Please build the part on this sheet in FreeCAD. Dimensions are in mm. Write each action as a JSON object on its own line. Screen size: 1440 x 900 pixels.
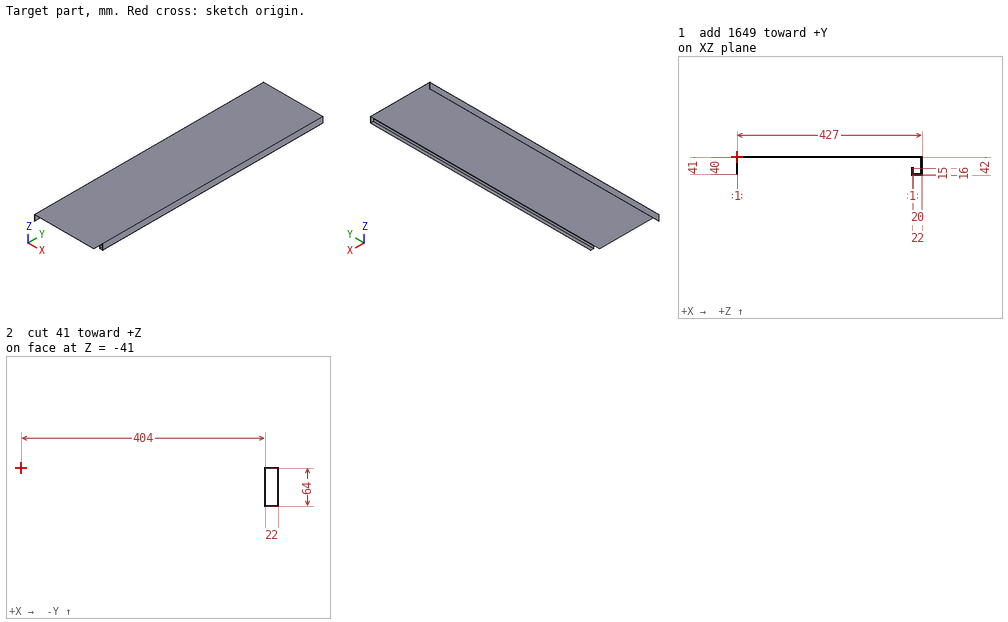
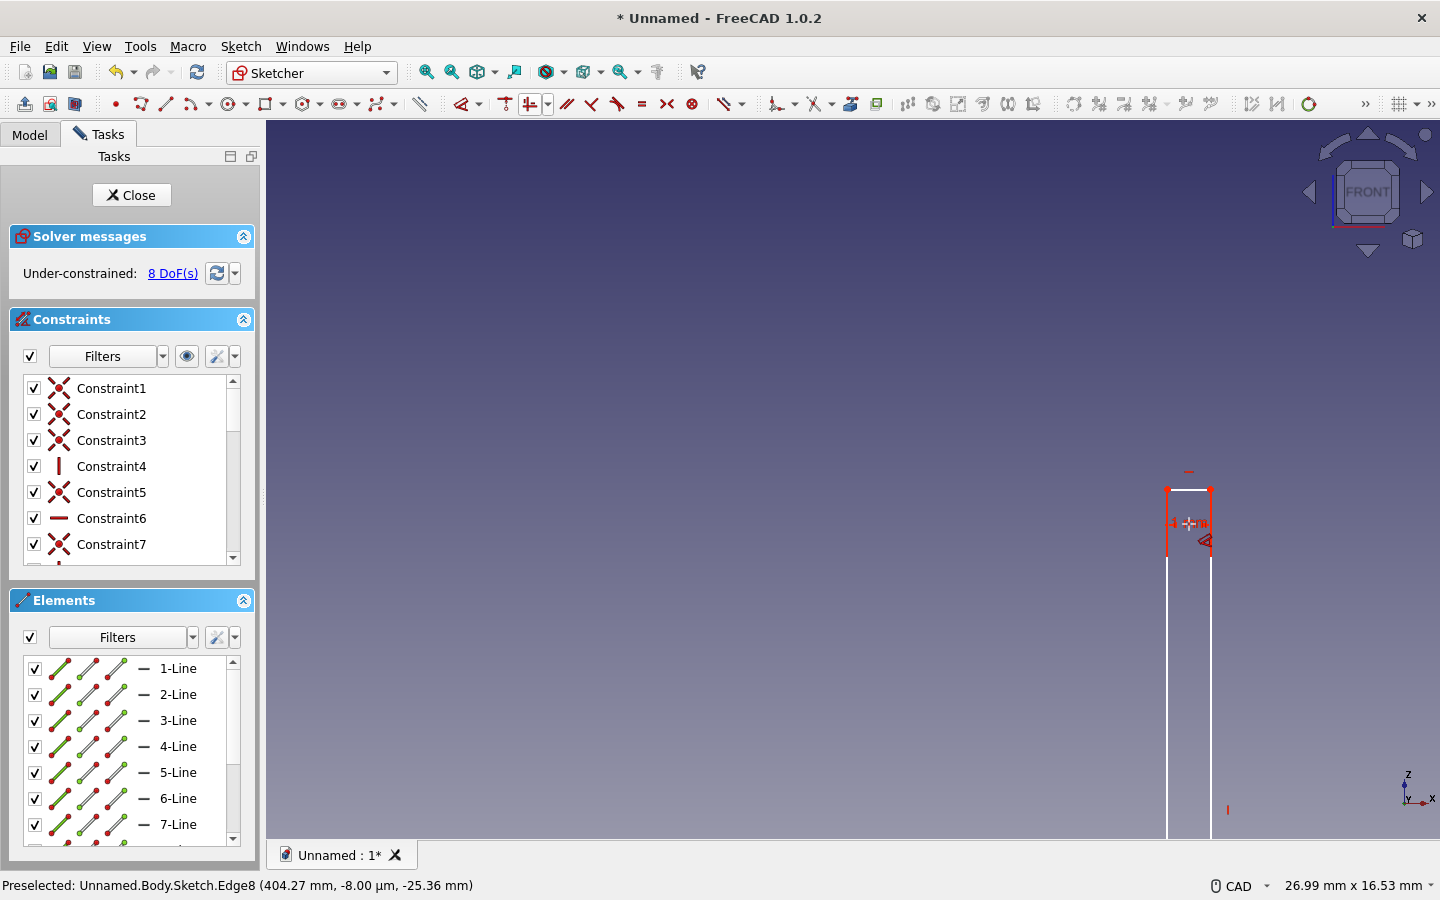
{"action": "scroll", "coordinate": [1201, 491], "scroll_direction": "down", "scroll_amount": 15}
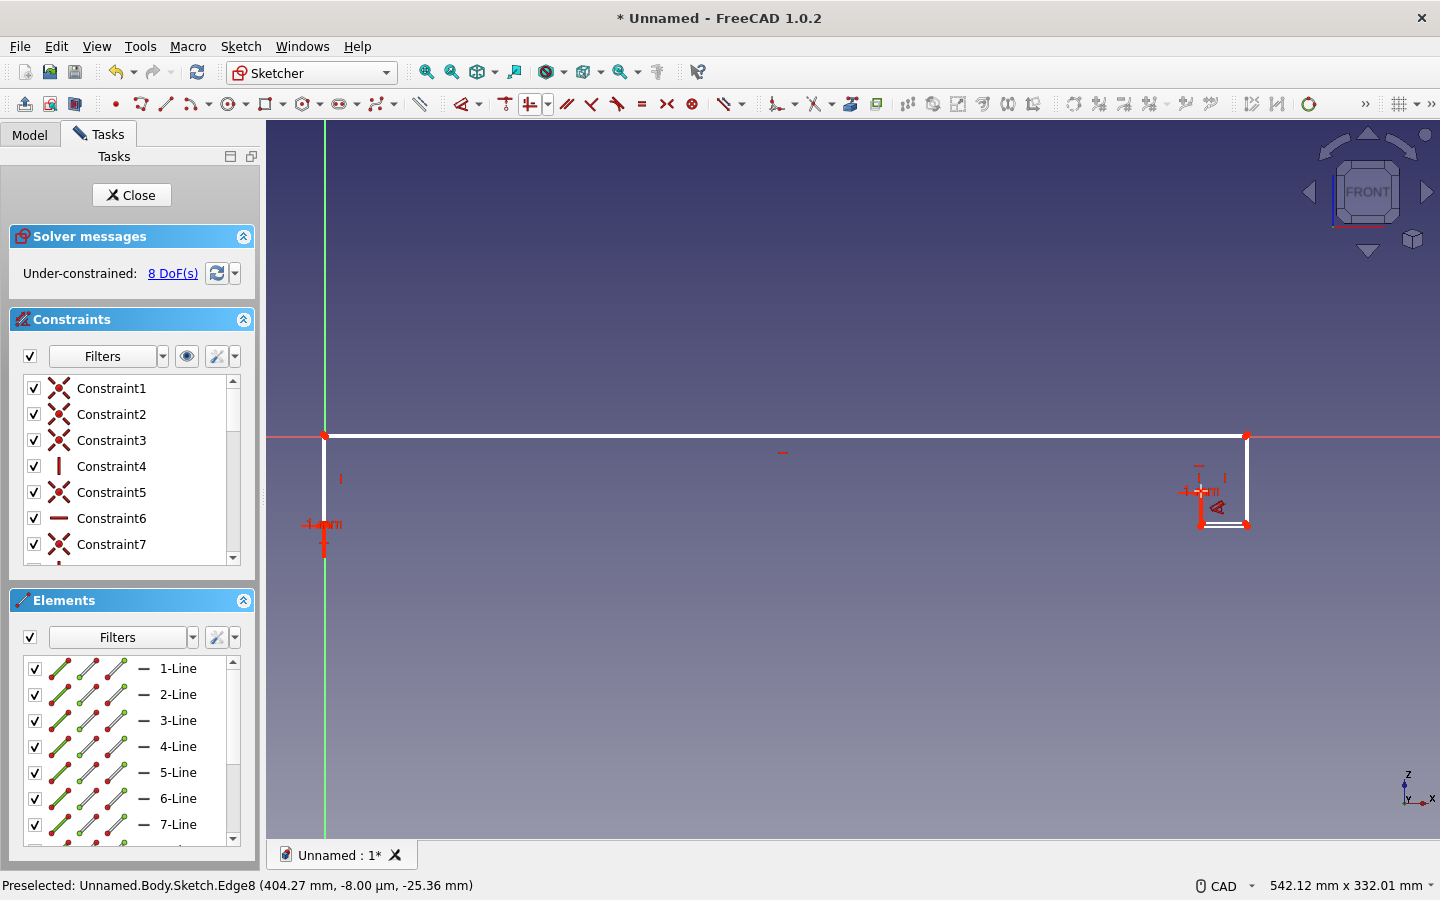
{"action": "scroll", "coordinate": [325, 463], "scroll_direction": "up", "scroll_amount": 10}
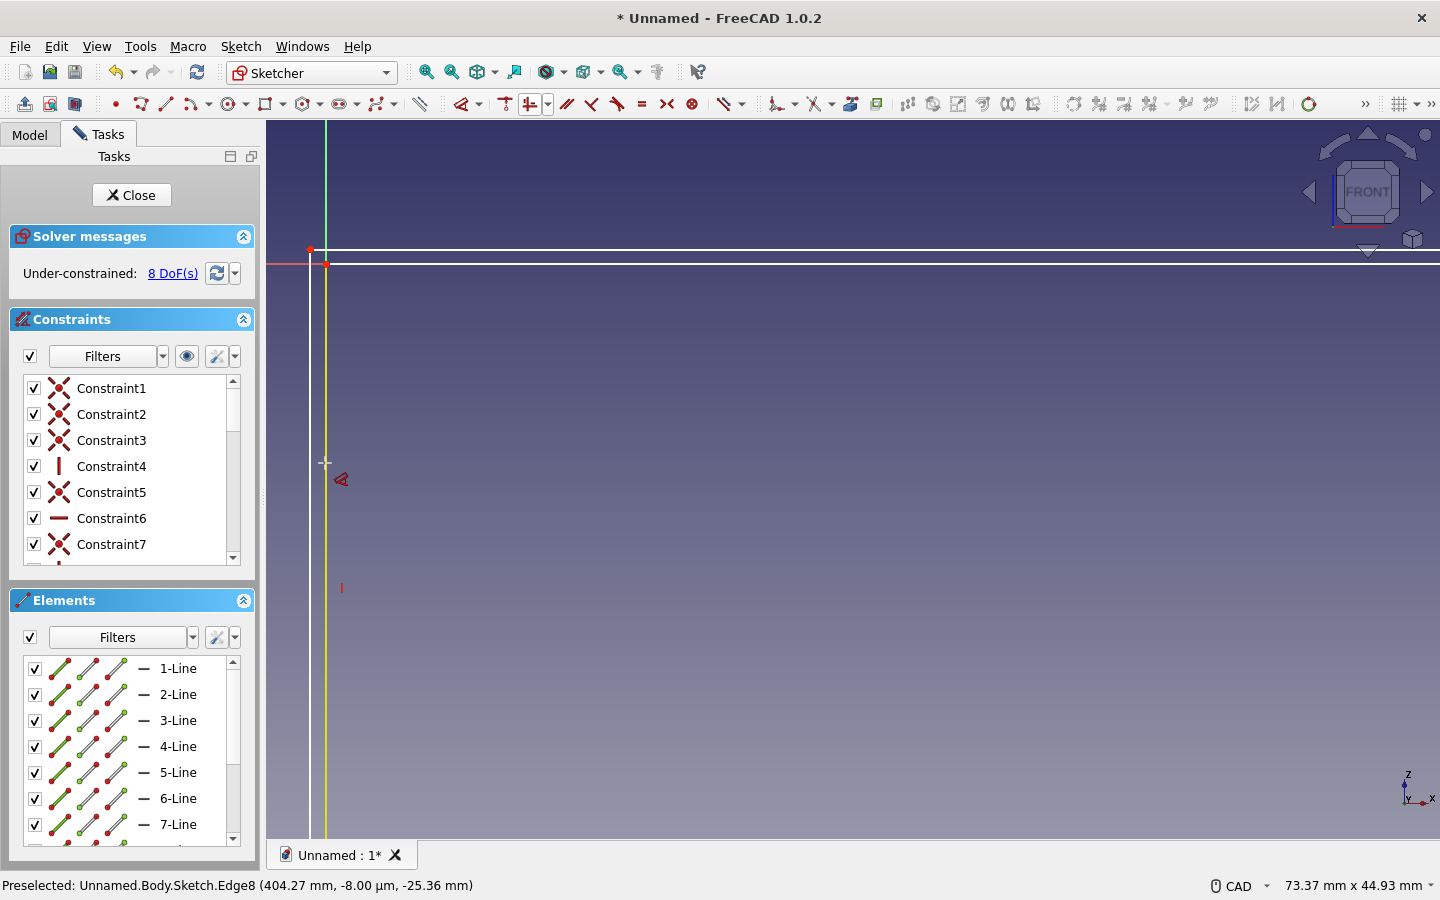
{"action": "left_click", "coordinate": [326, 459]}
{"action": "left_click", "coordinate": [360, 538]}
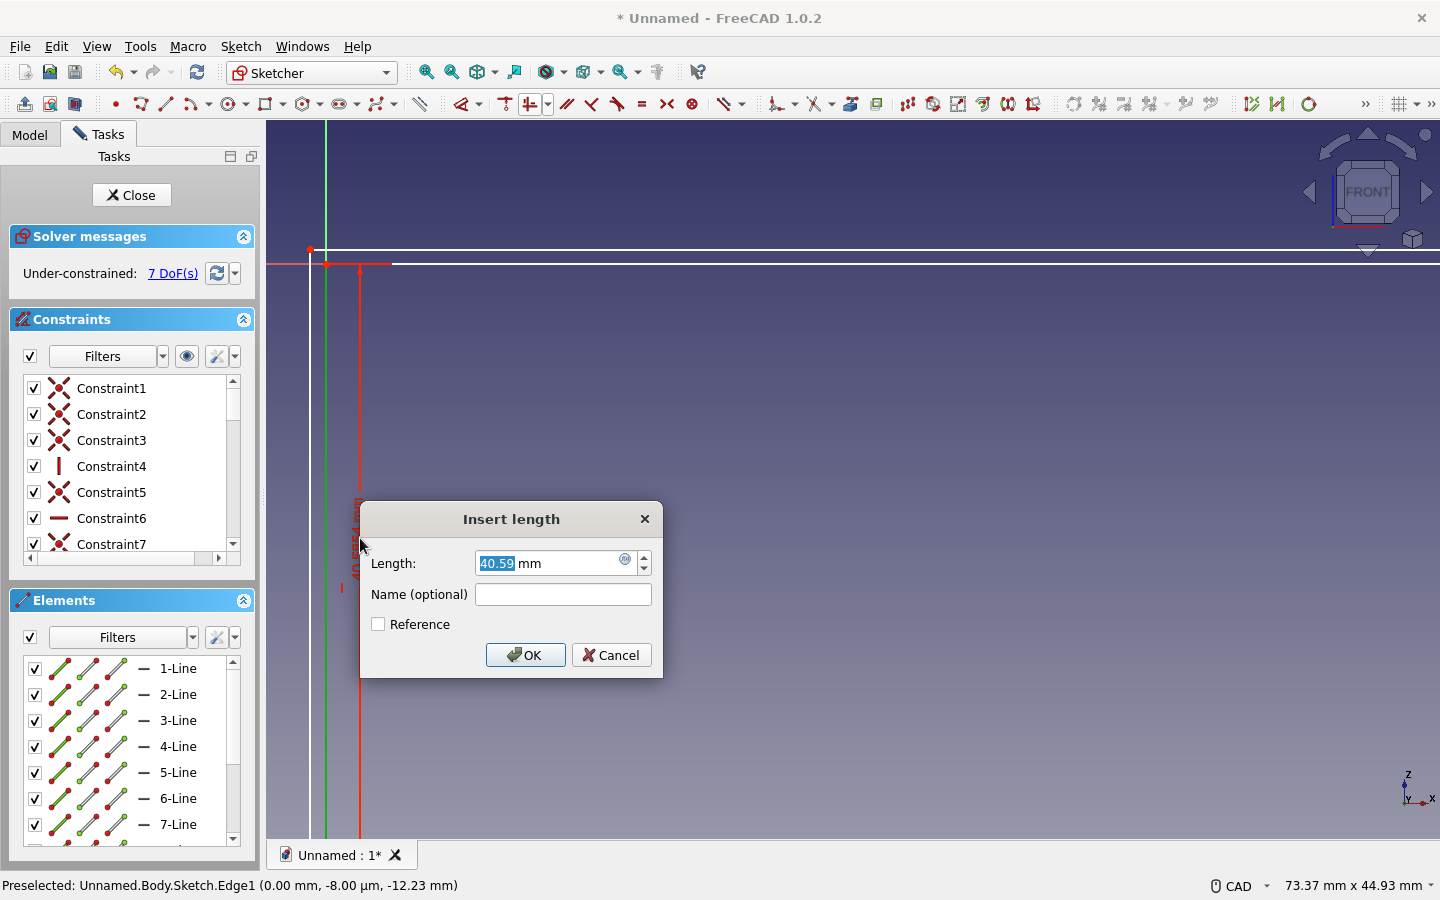
{"action": "type", "text": "40"}
{"action": "key", "text": "Return"}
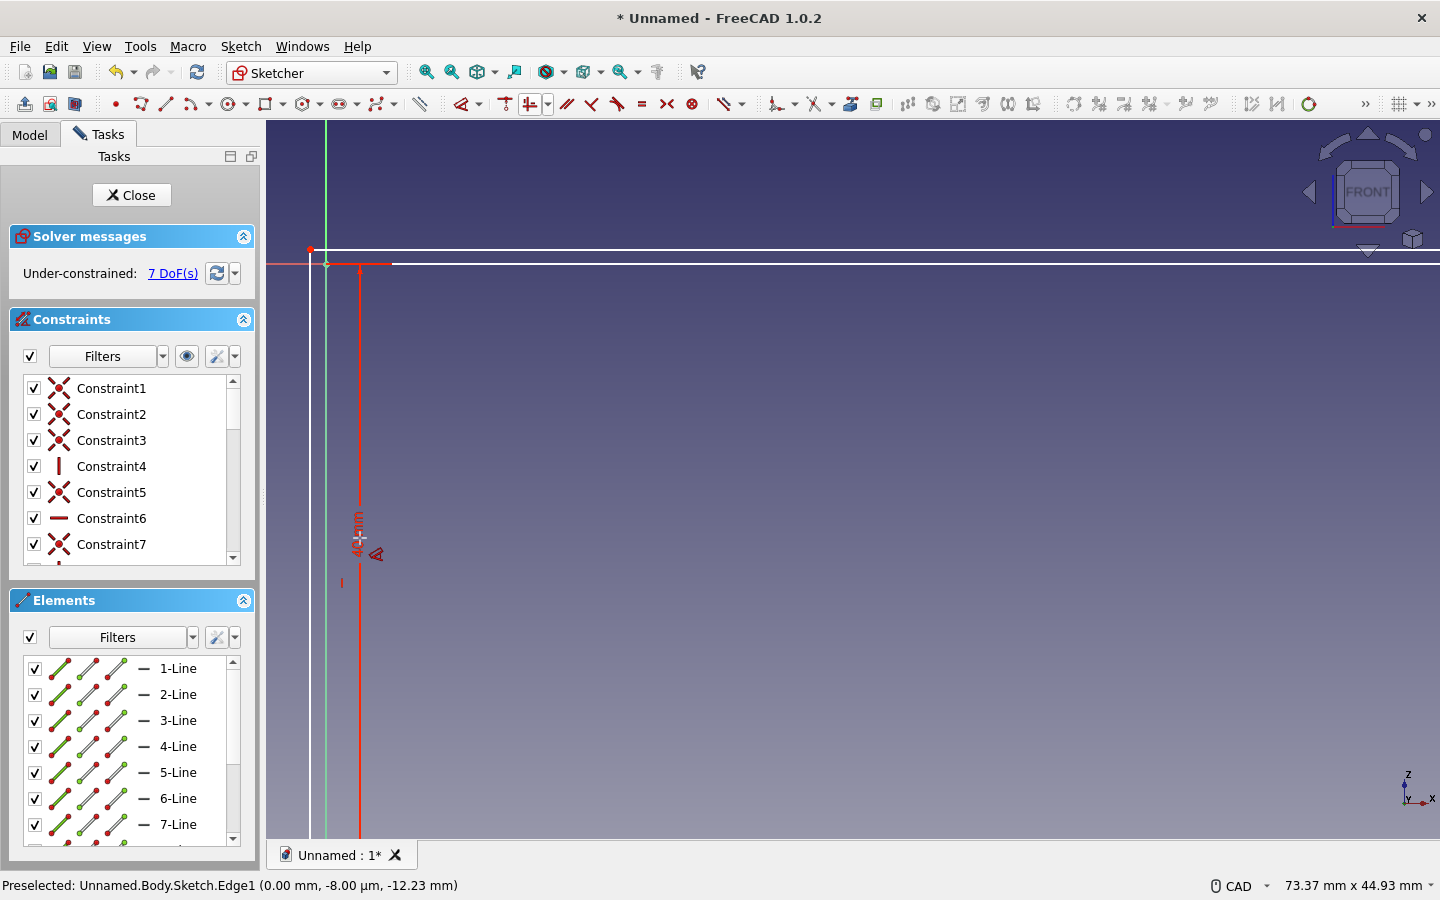
{"action": "left_click", "coordinate": [310, 708]}
{"action": "left_click", "coordinate": [344, 401]}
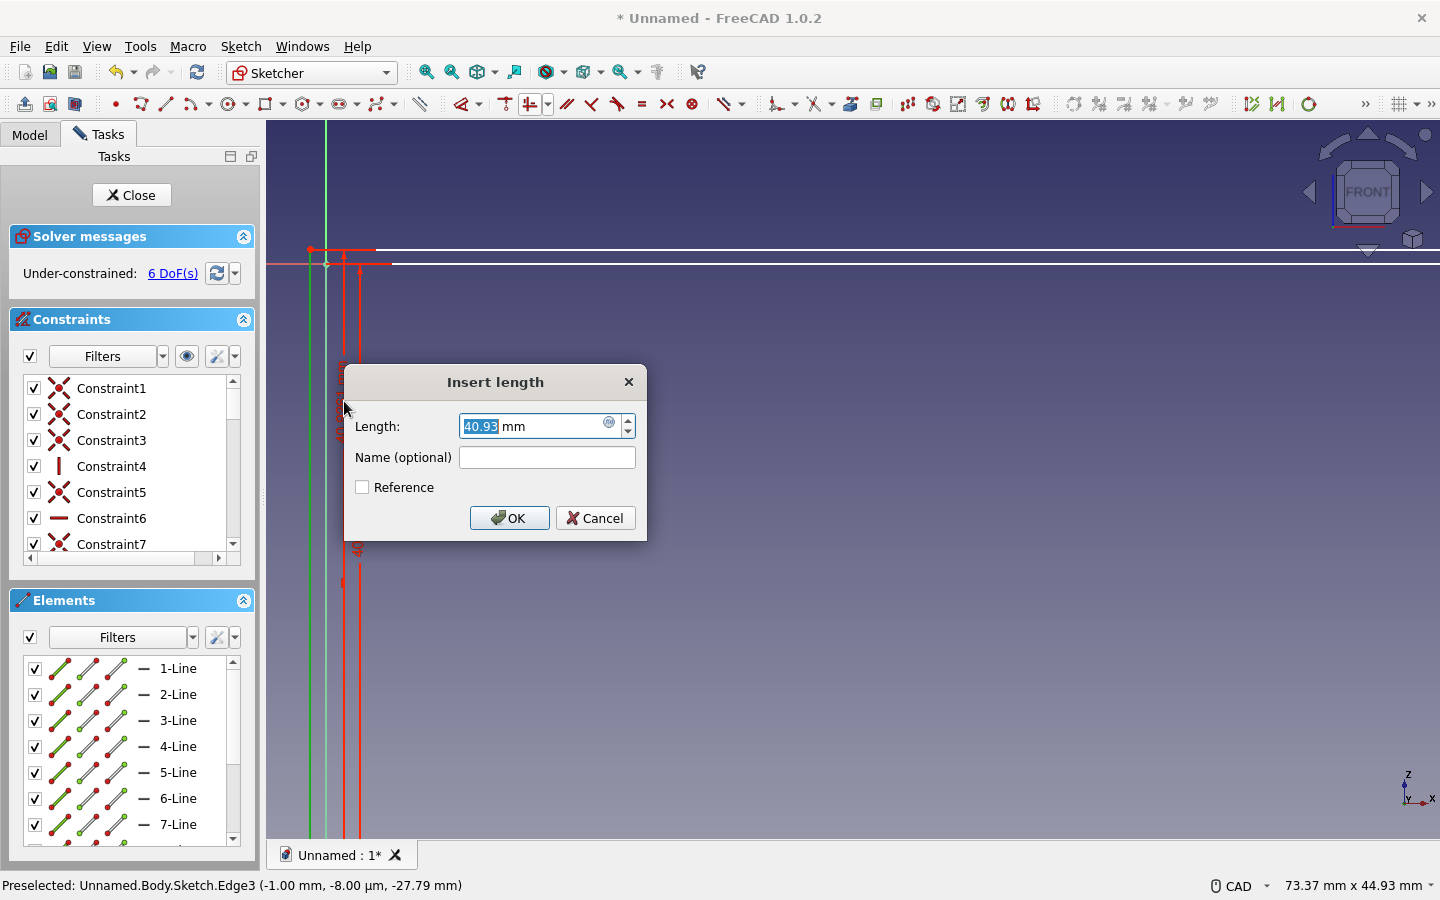
{"action": "type", "text": "41"}
{"action": "key", "text": "Return"}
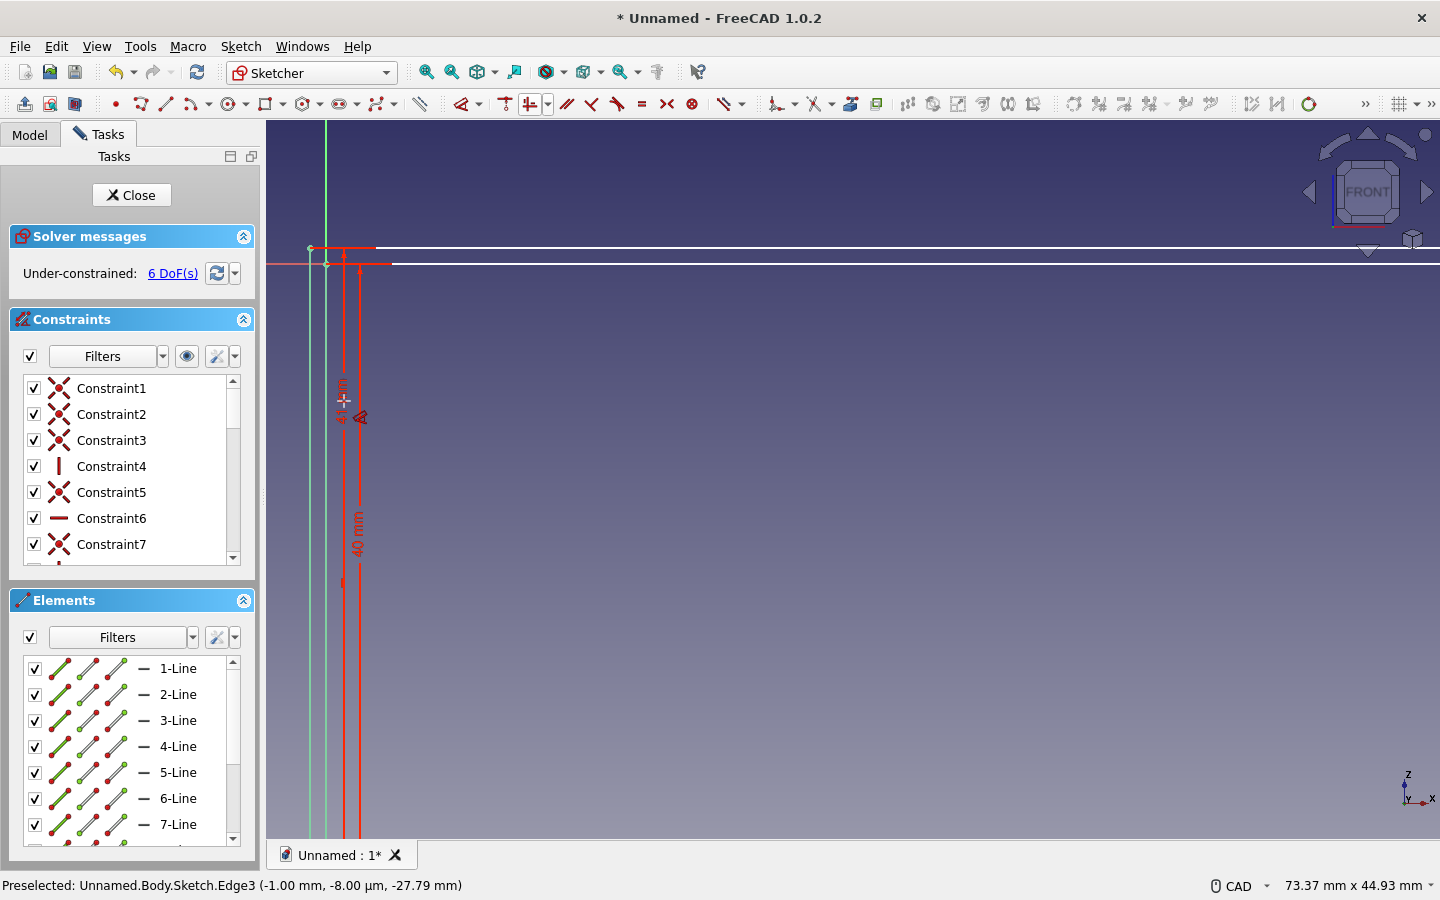
{"action": "scroll", "coordinate": [418, 466], "scroll_direction": "down", "scroll_amount": 11}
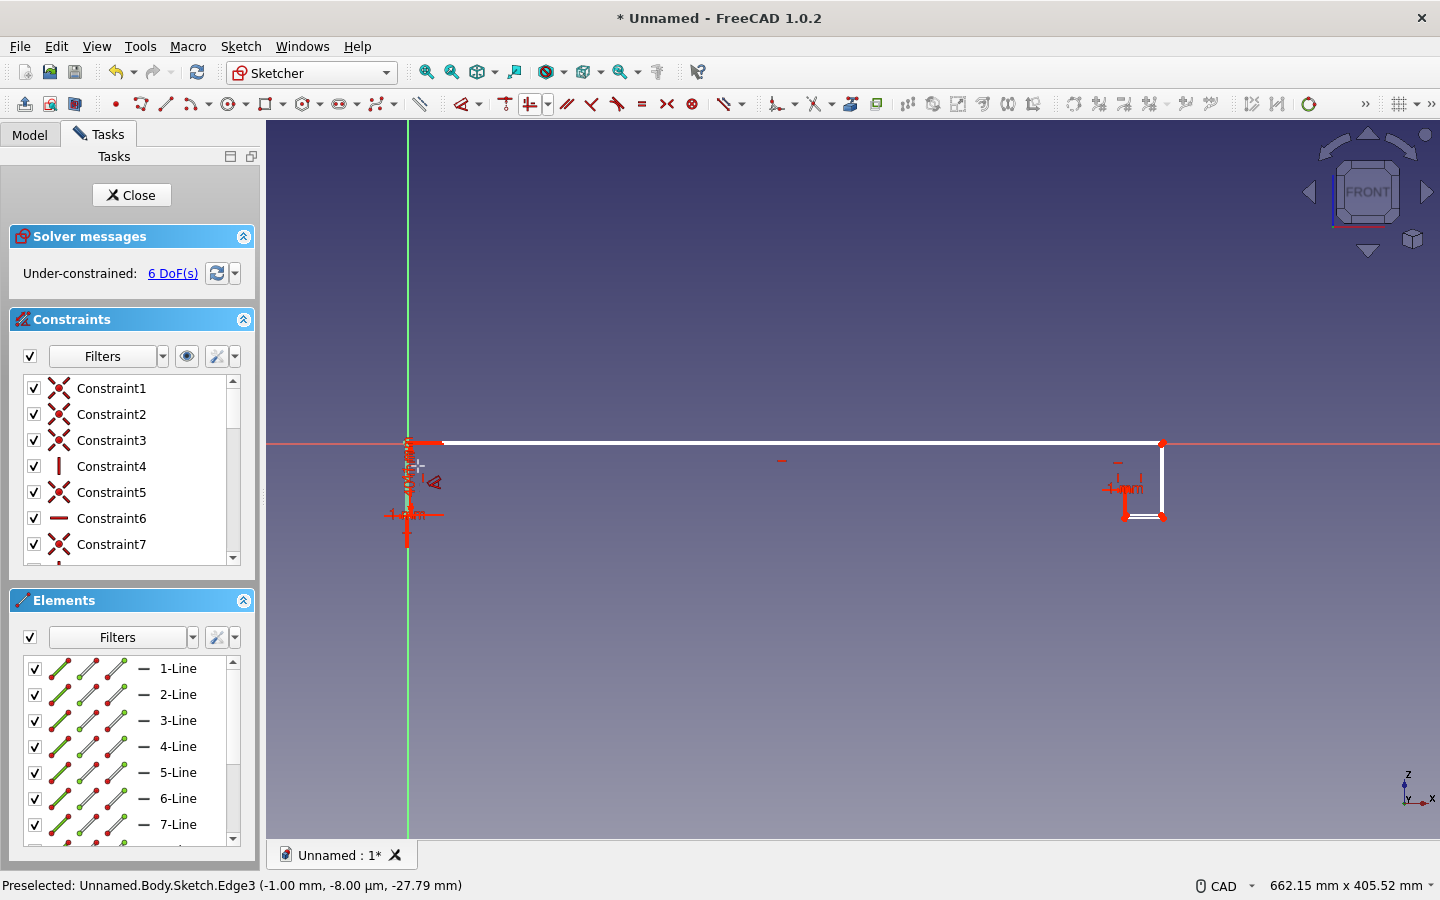
{"action": "scroll", "coordinate": [1163, 465], "scroll_direction": "up", "scroll_amount": 11}